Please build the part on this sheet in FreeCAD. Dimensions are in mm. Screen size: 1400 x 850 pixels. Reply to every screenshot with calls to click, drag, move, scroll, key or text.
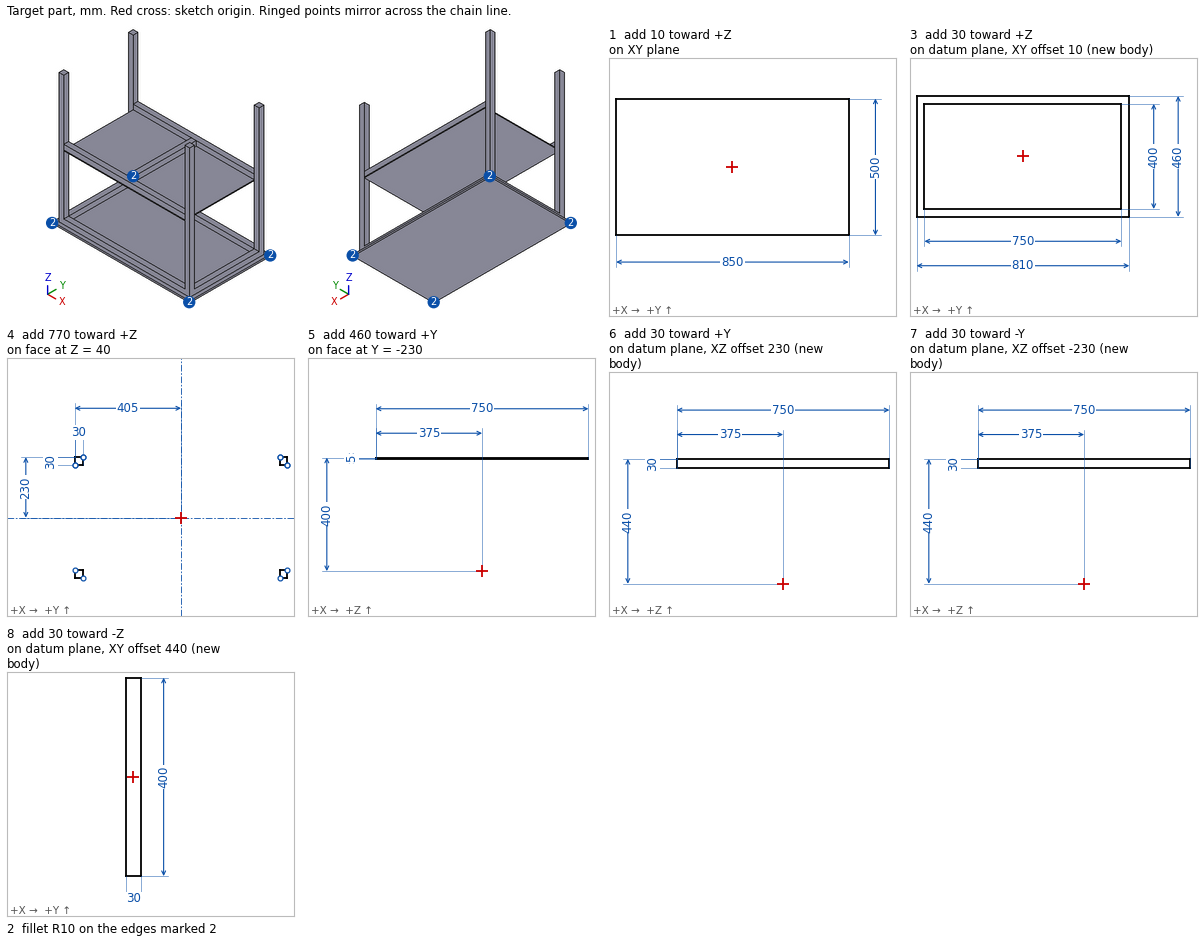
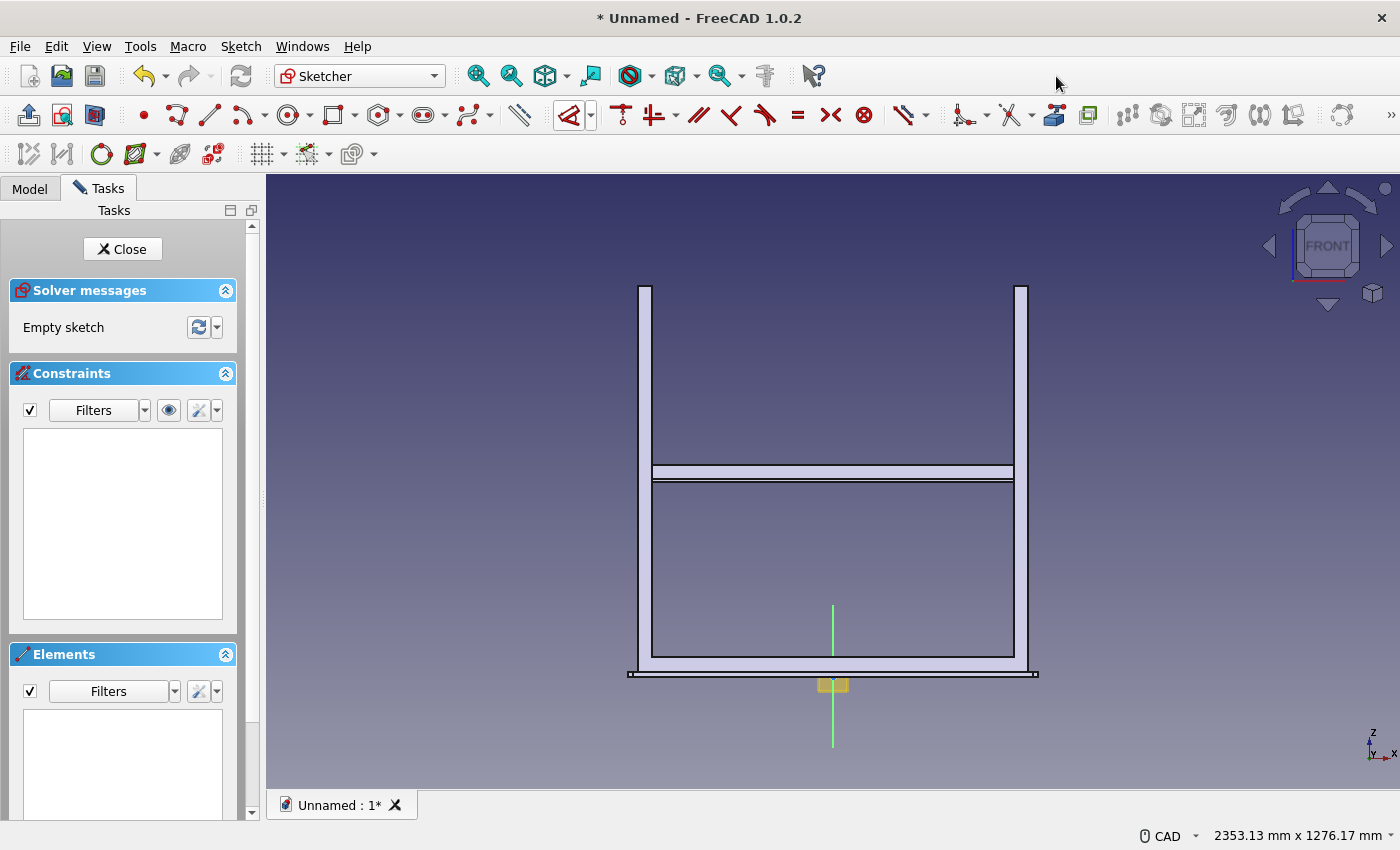
scroll(916, 679, up, 3)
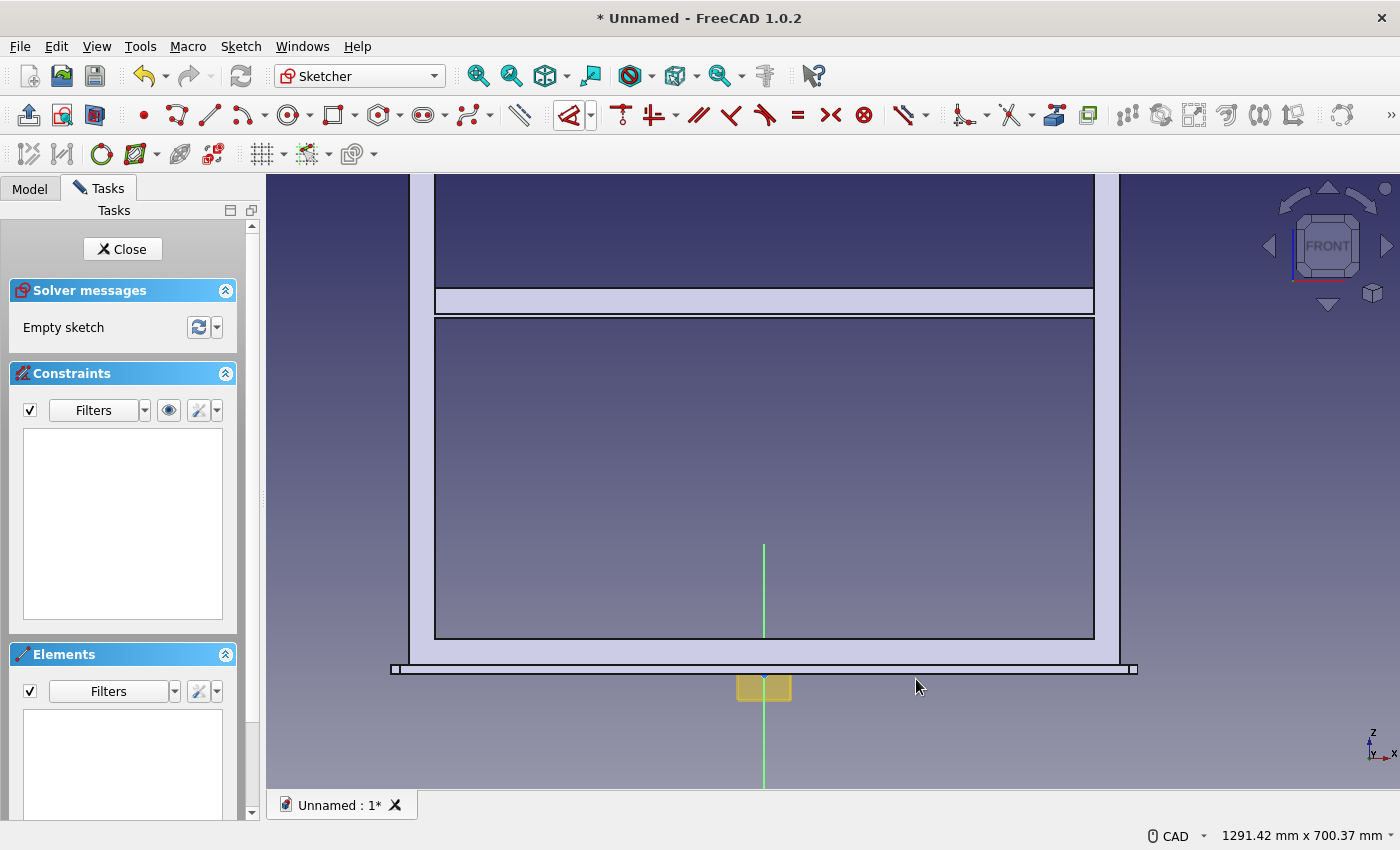
click(332, 116)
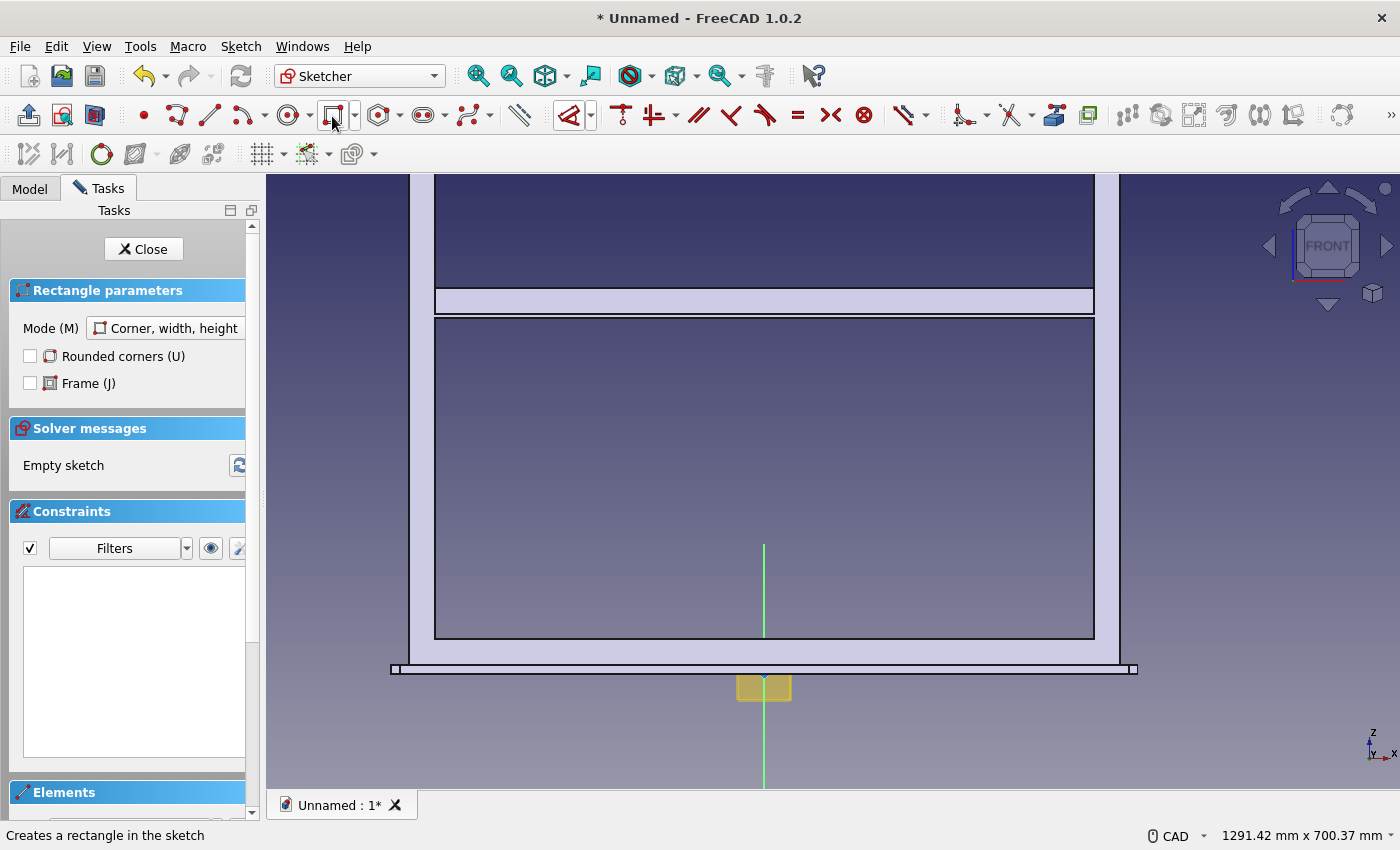
click(435, 288)
click(1094, 314)
key(Escape)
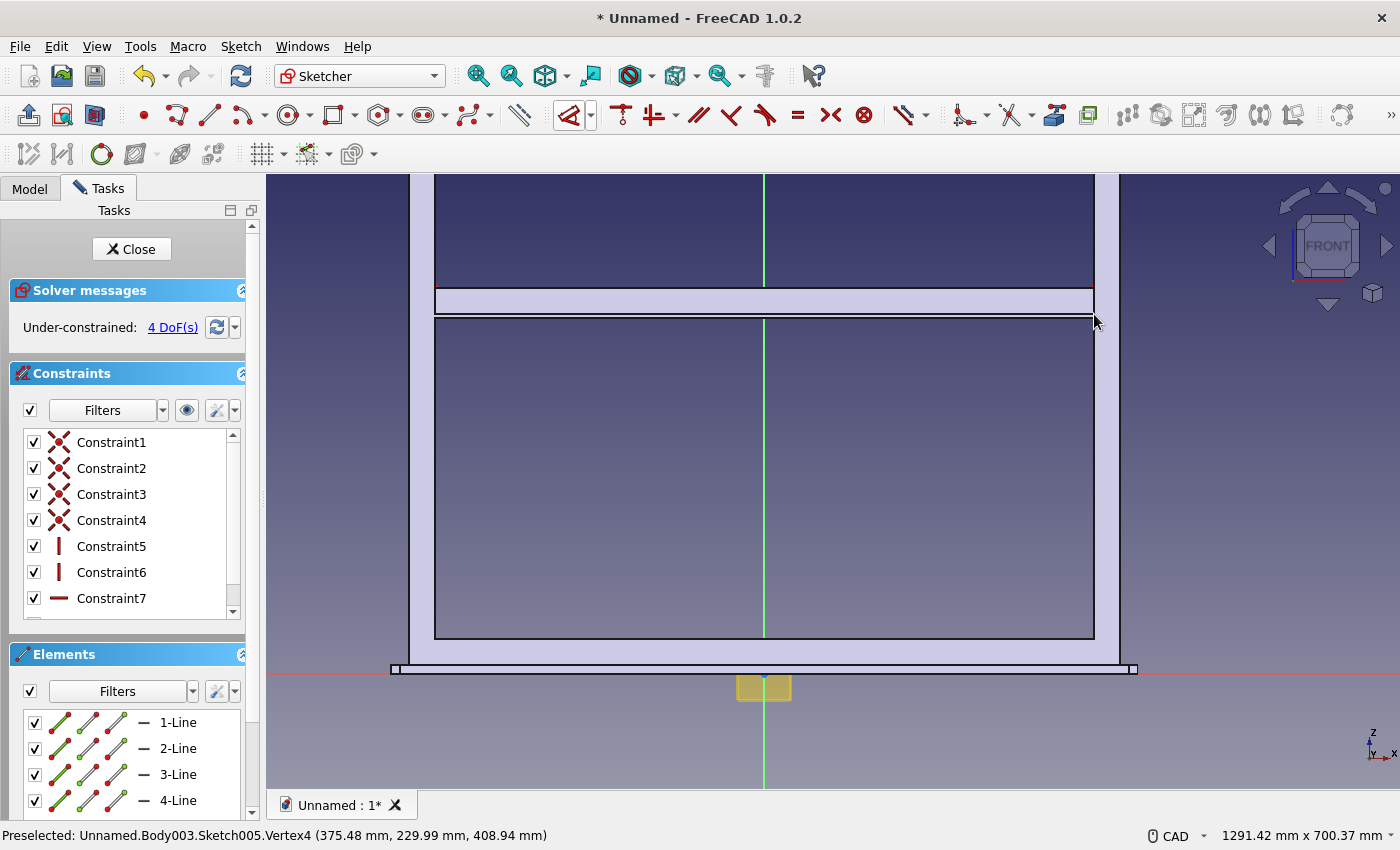
scroll(435, 299, up, 3)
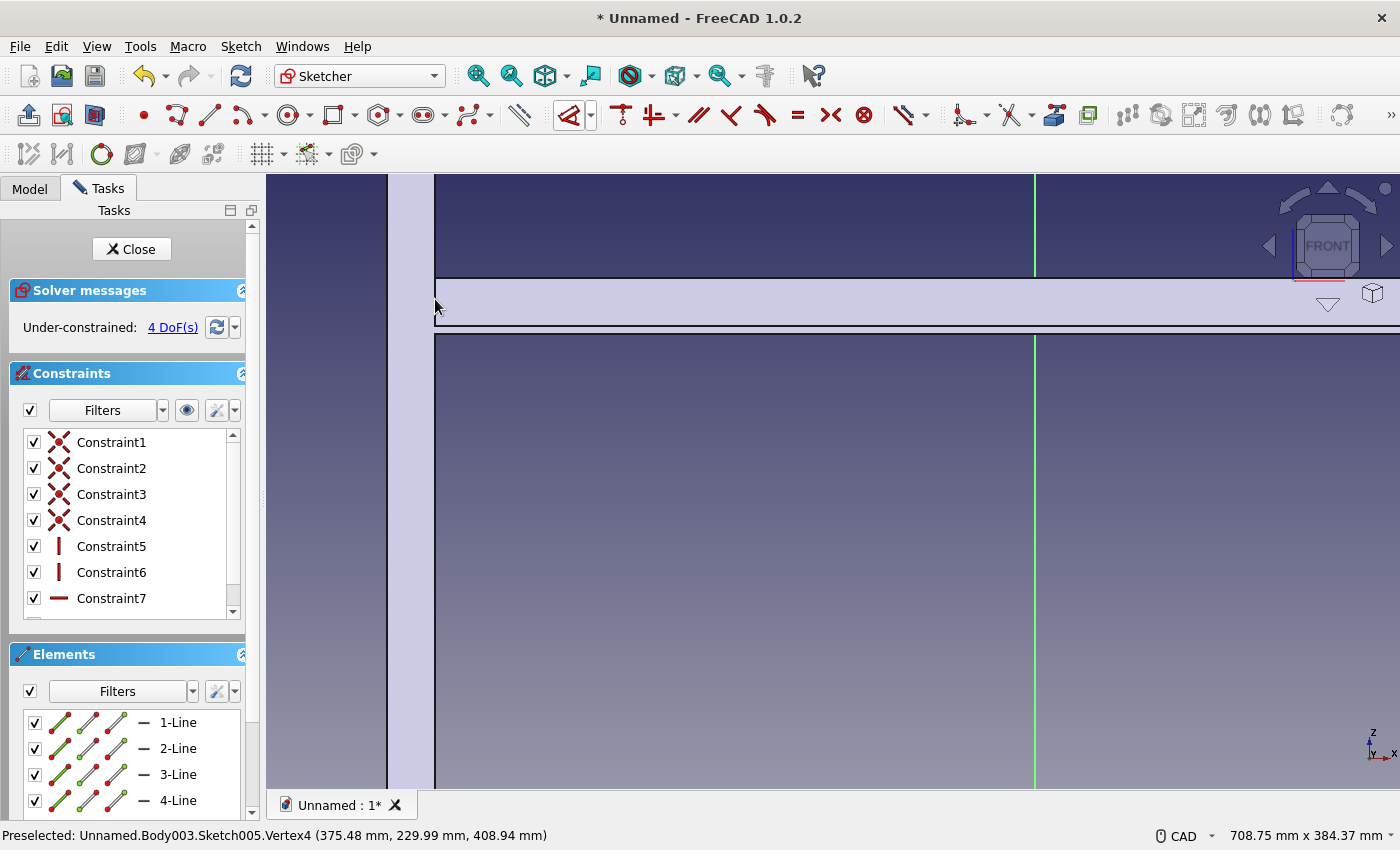
click(435, 300)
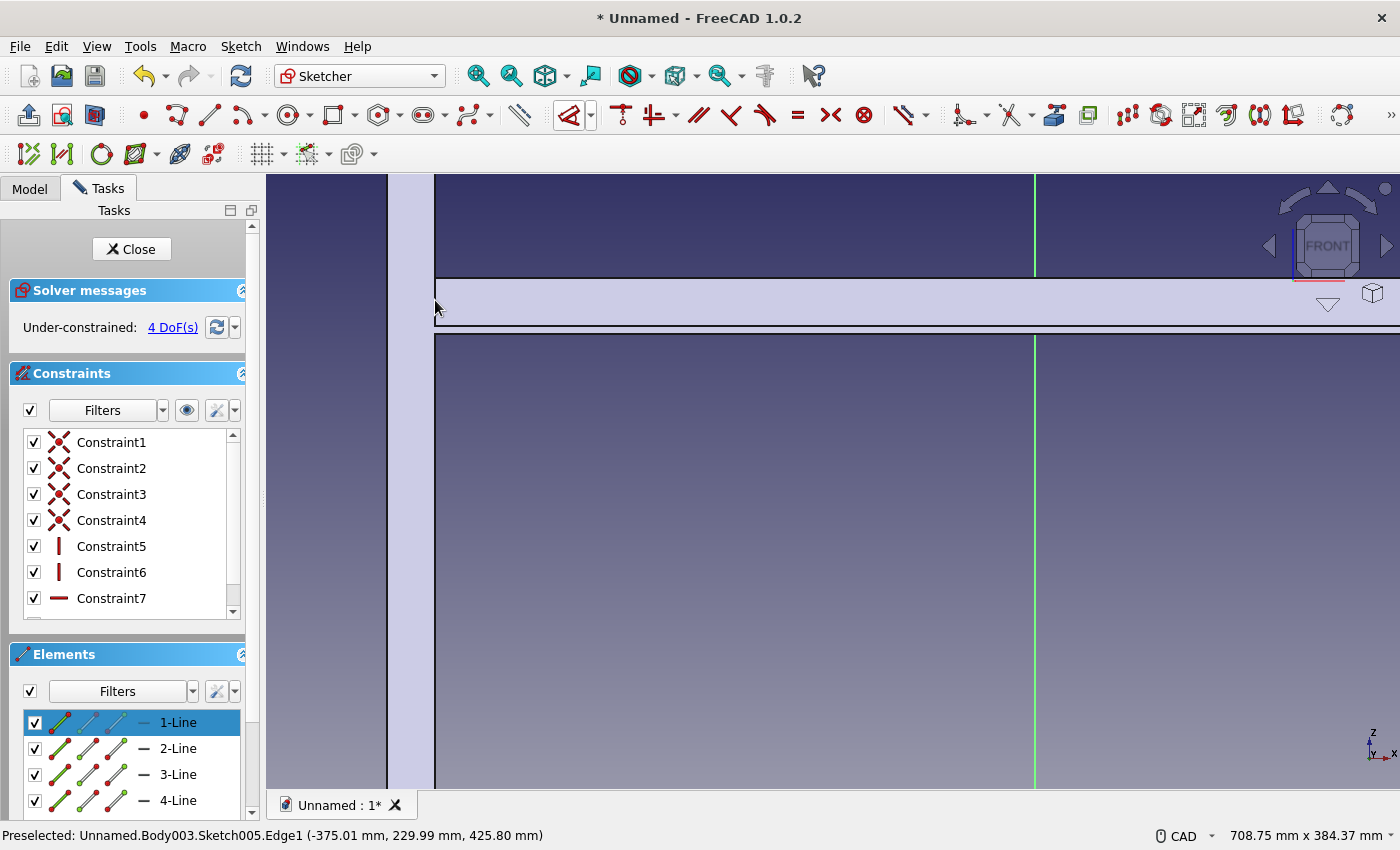
key(i)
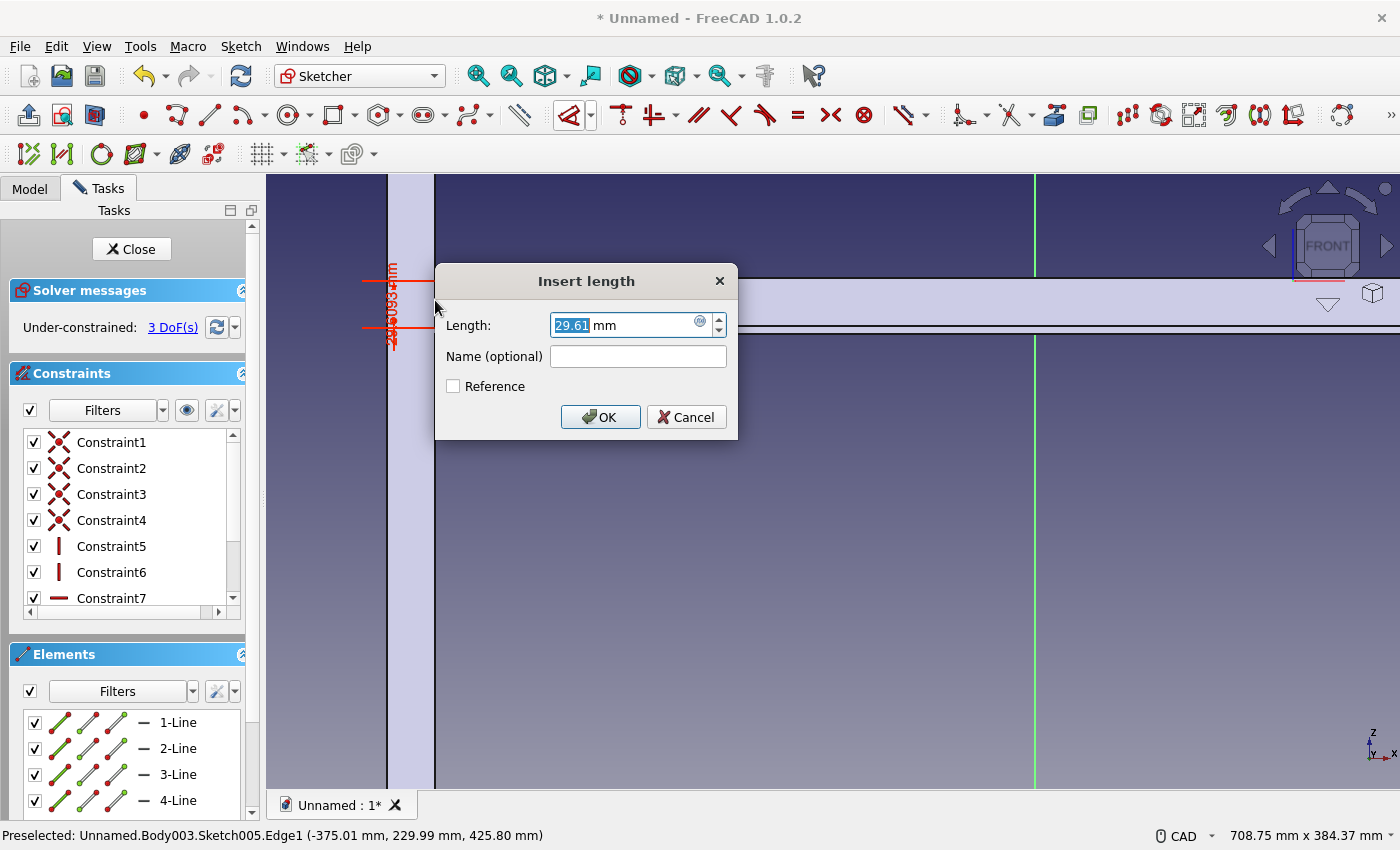
text(30)
key(Return)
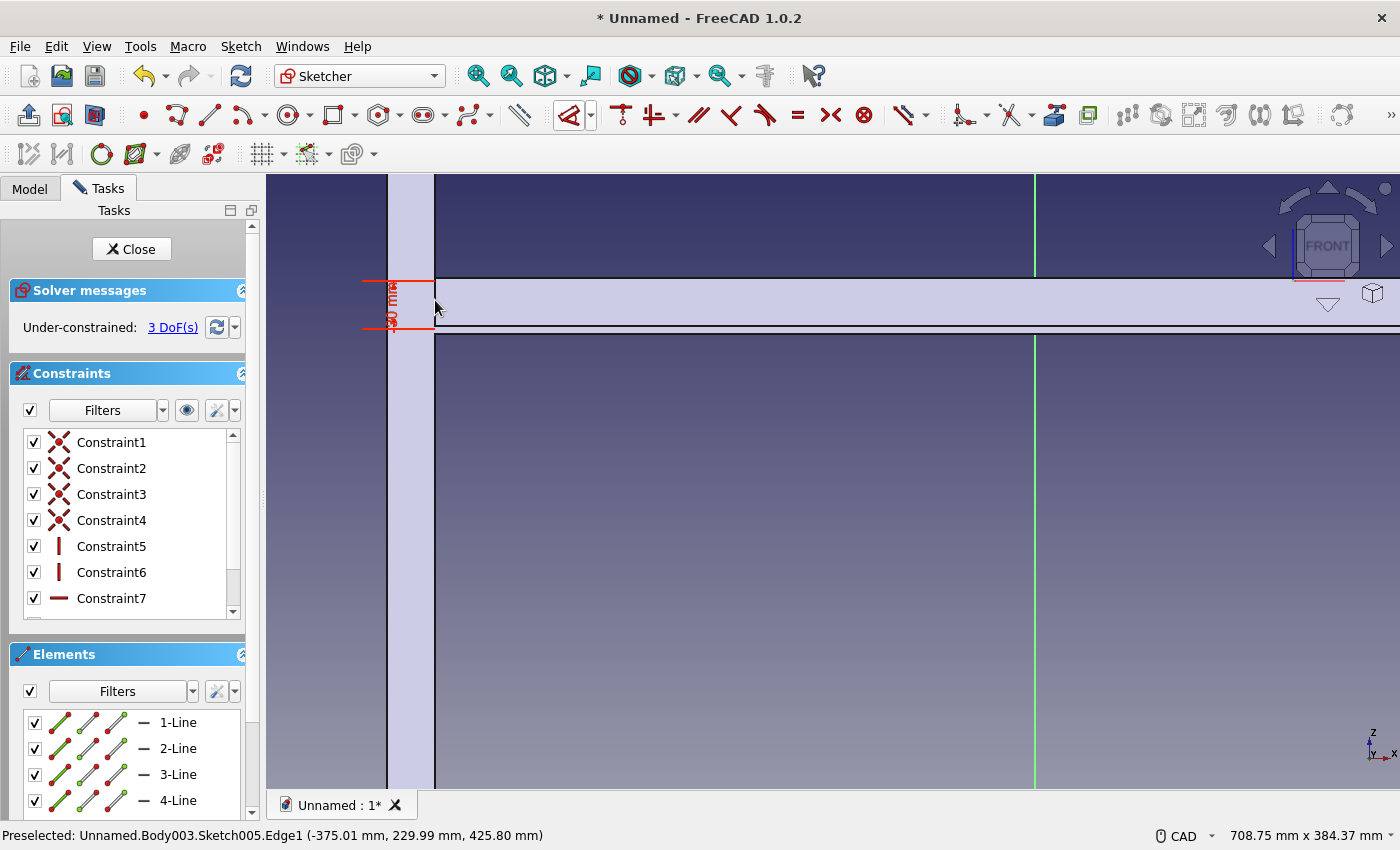
click(795, 328)